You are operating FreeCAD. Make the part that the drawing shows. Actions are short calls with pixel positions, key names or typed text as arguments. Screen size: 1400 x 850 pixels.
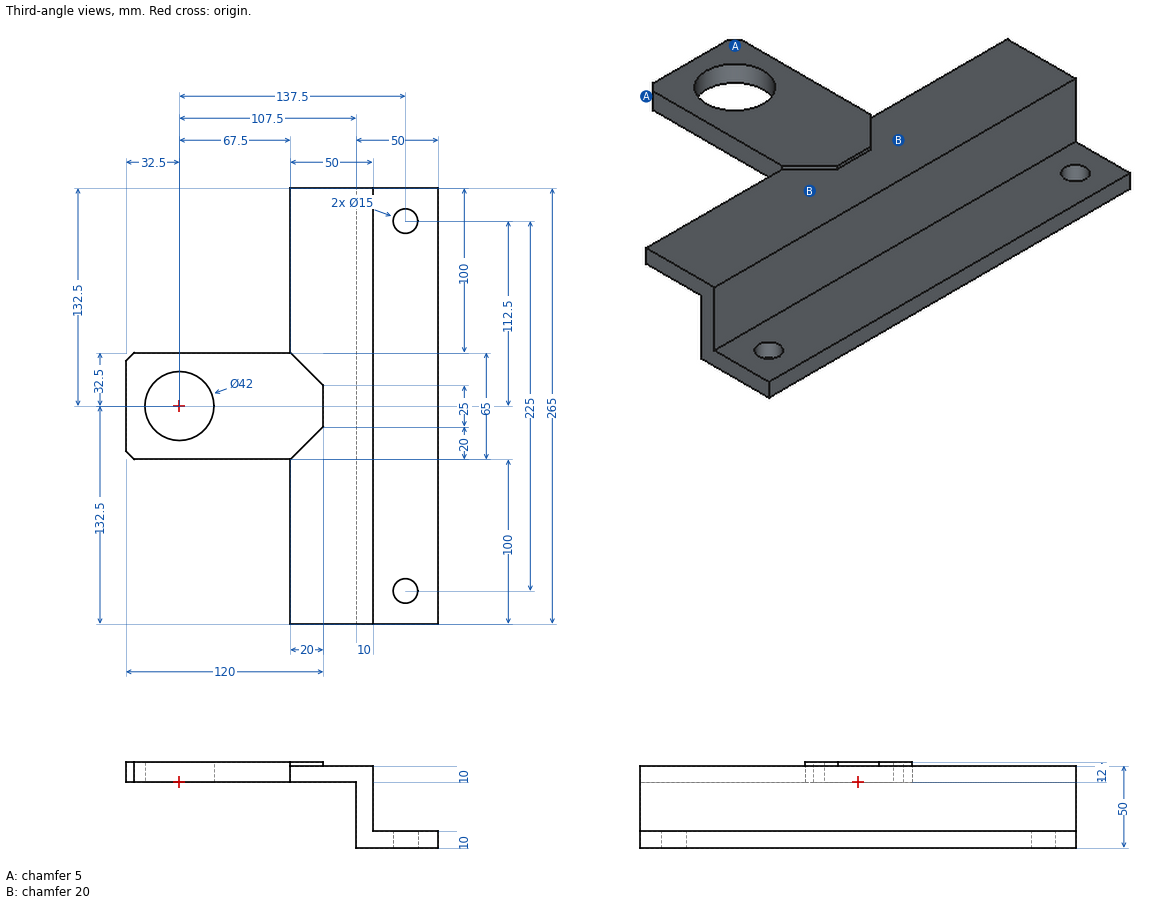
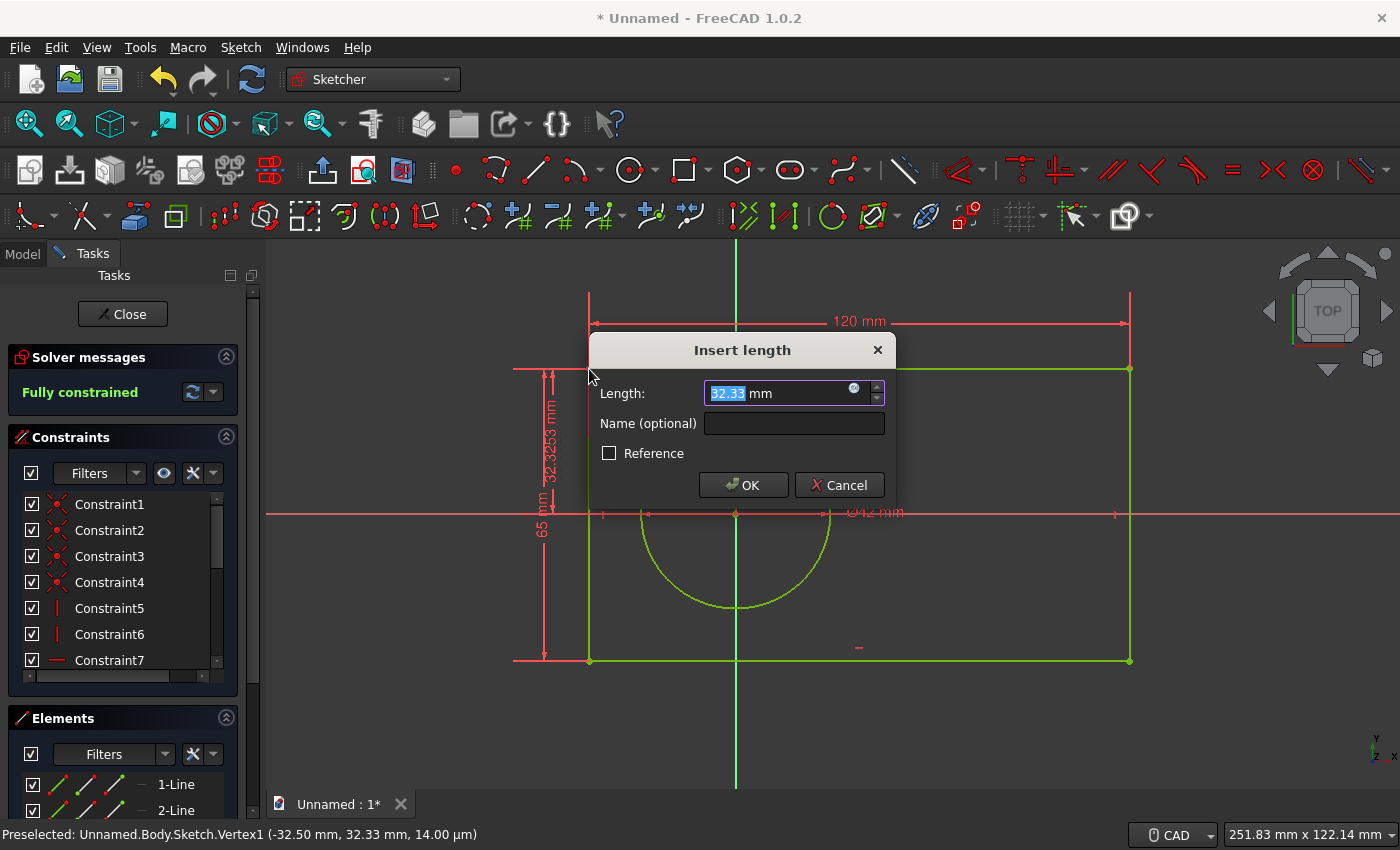
text(32.5)
key(Return)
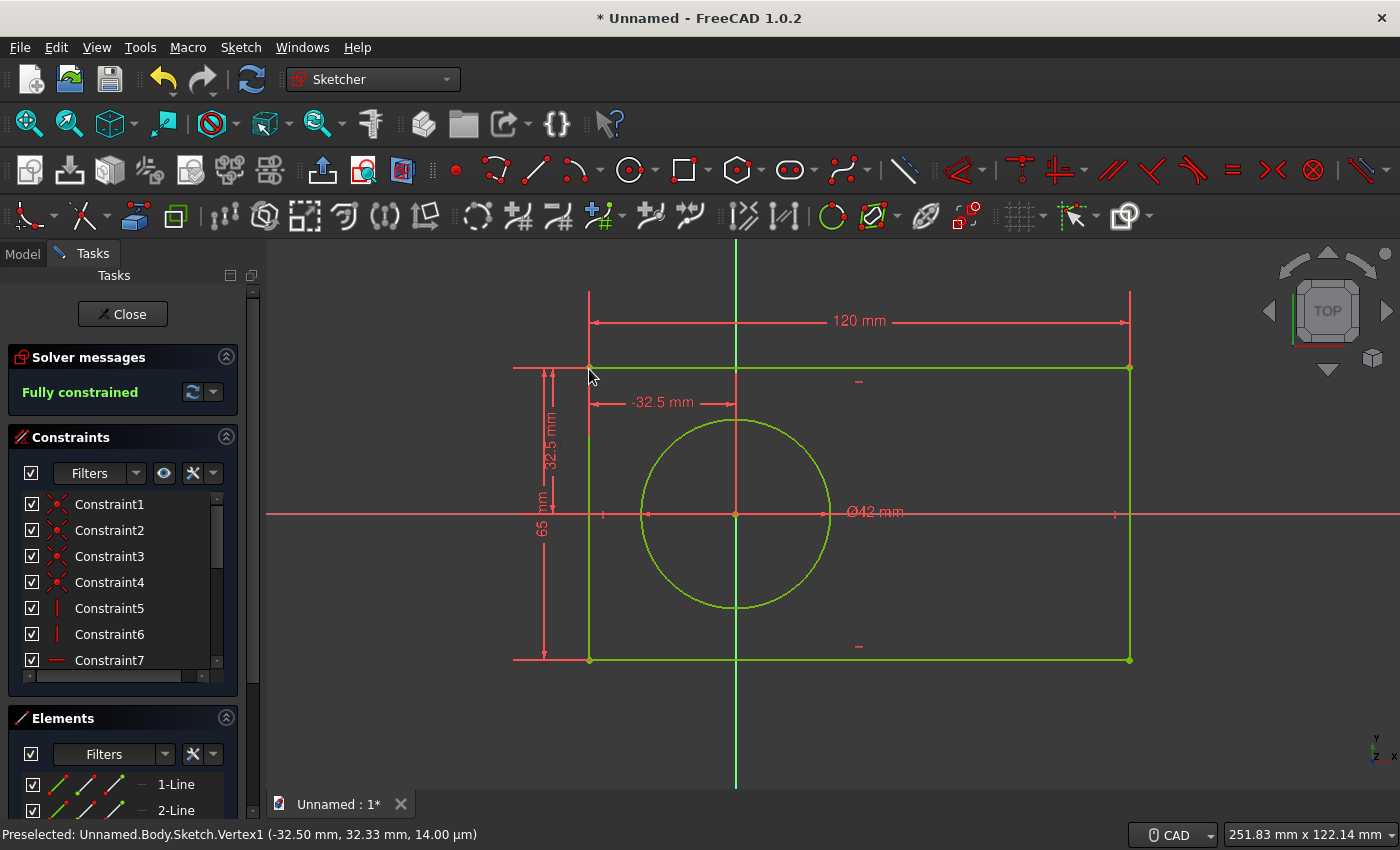
click(123, 314)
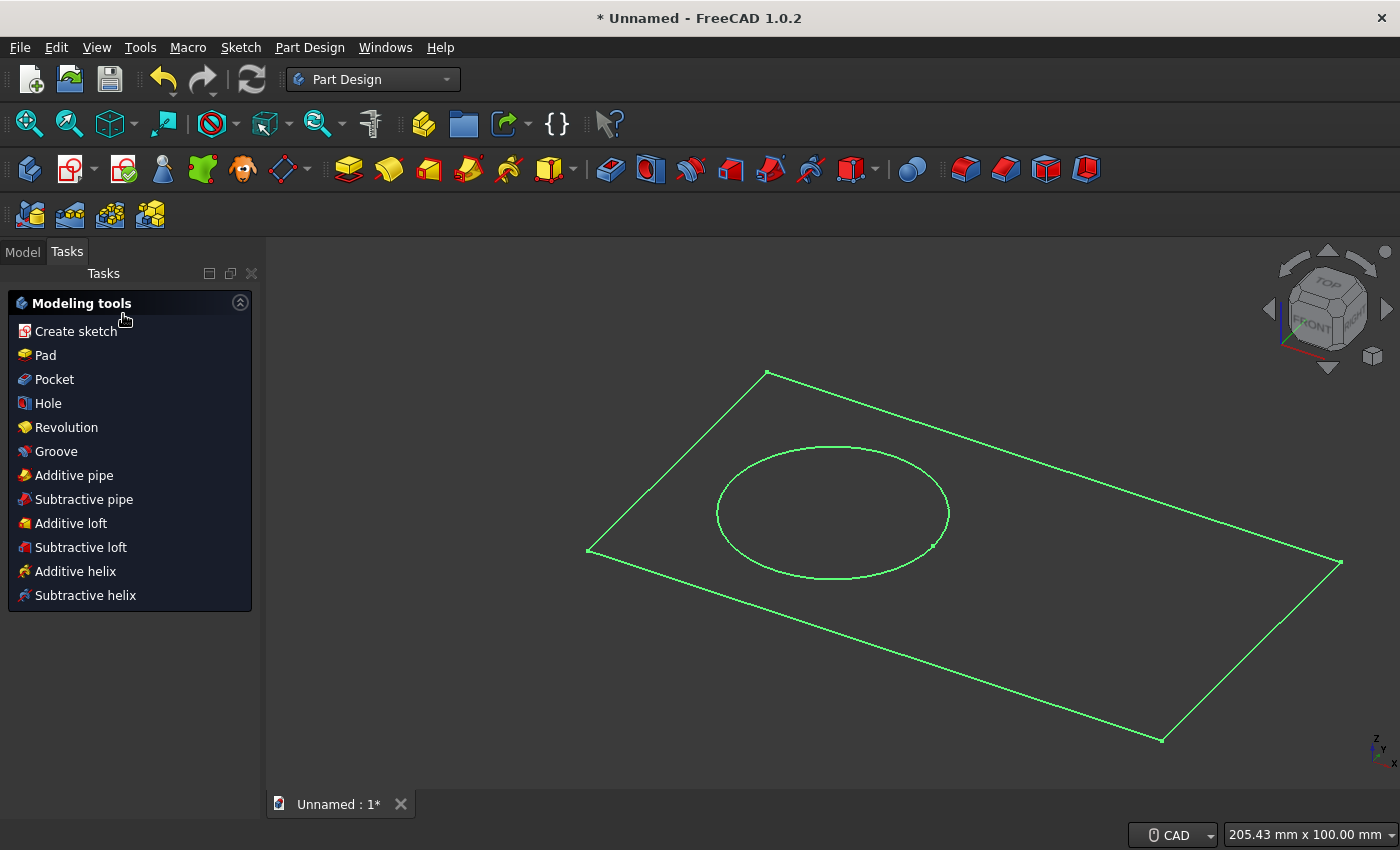
click(350, 170)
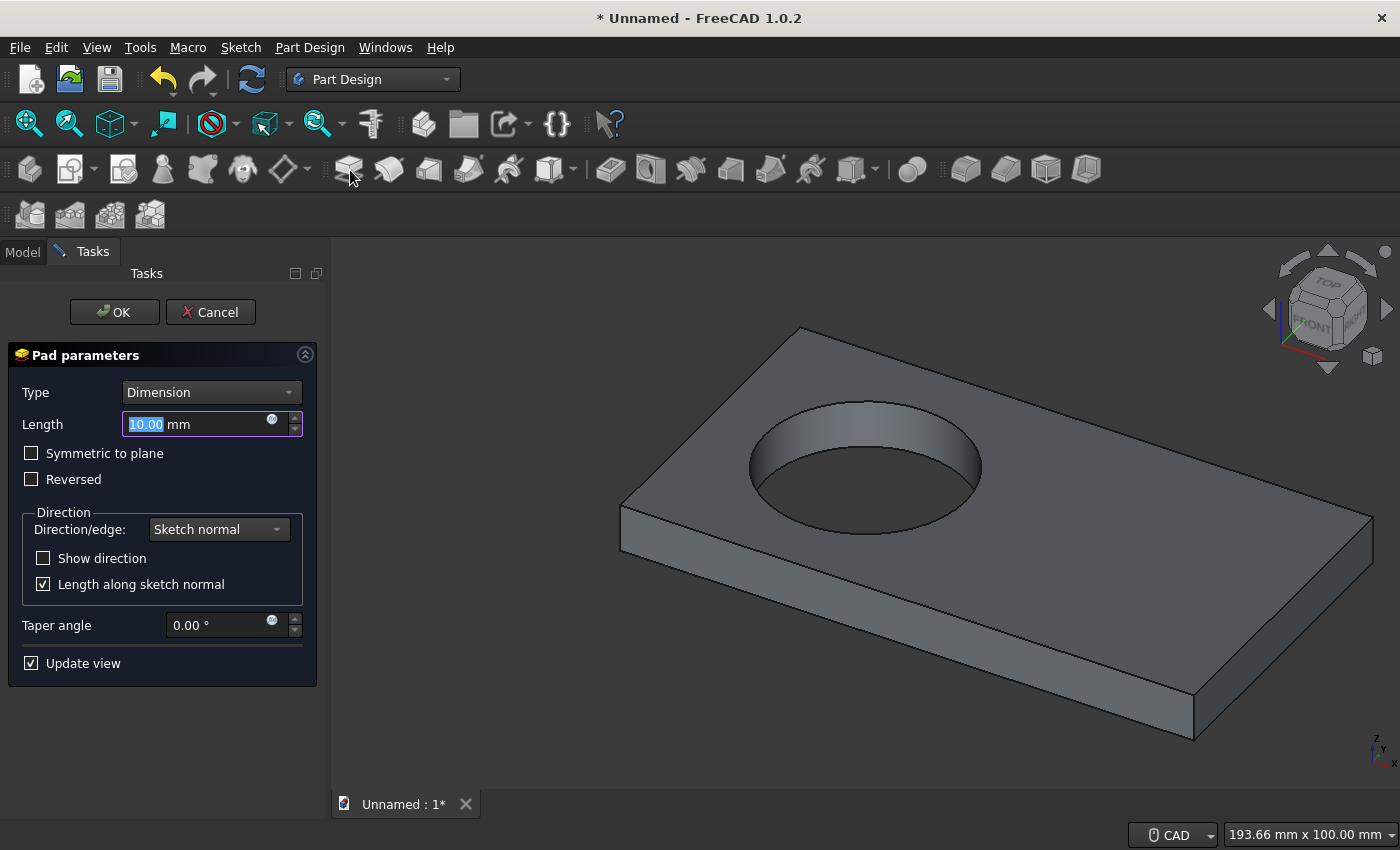
text(12)
key(Tab)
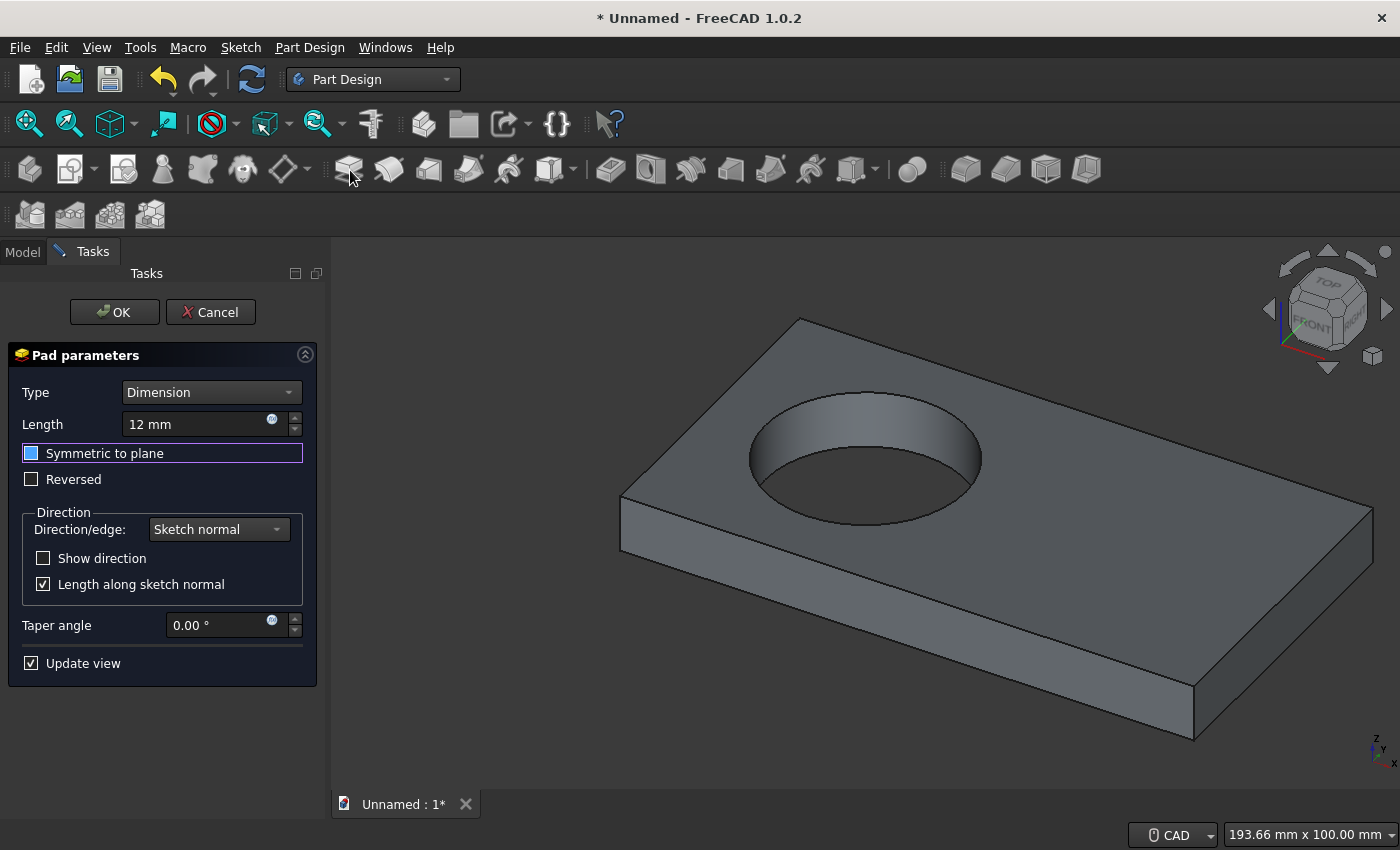
click(115, 312)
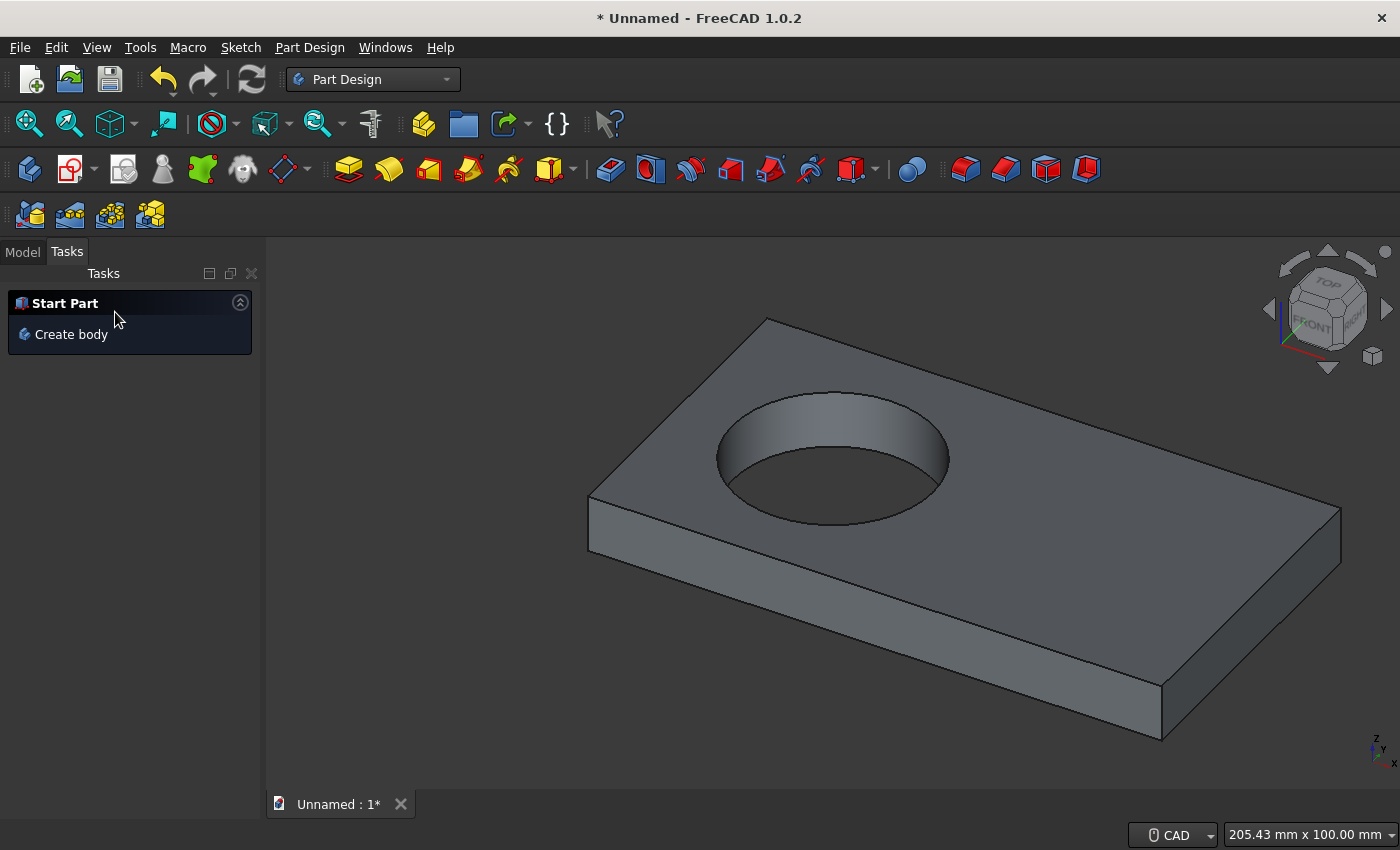
key(0)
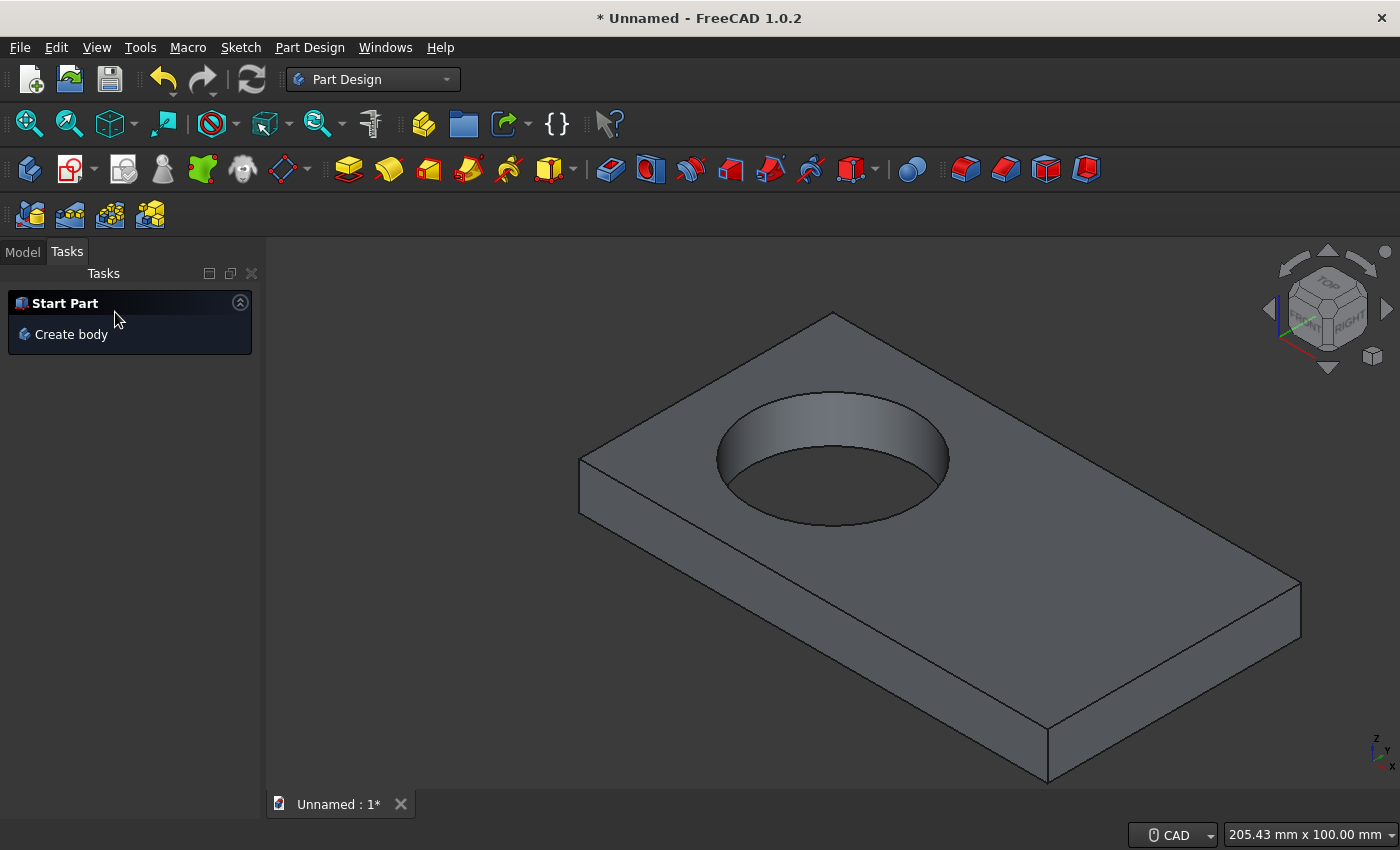
key(2)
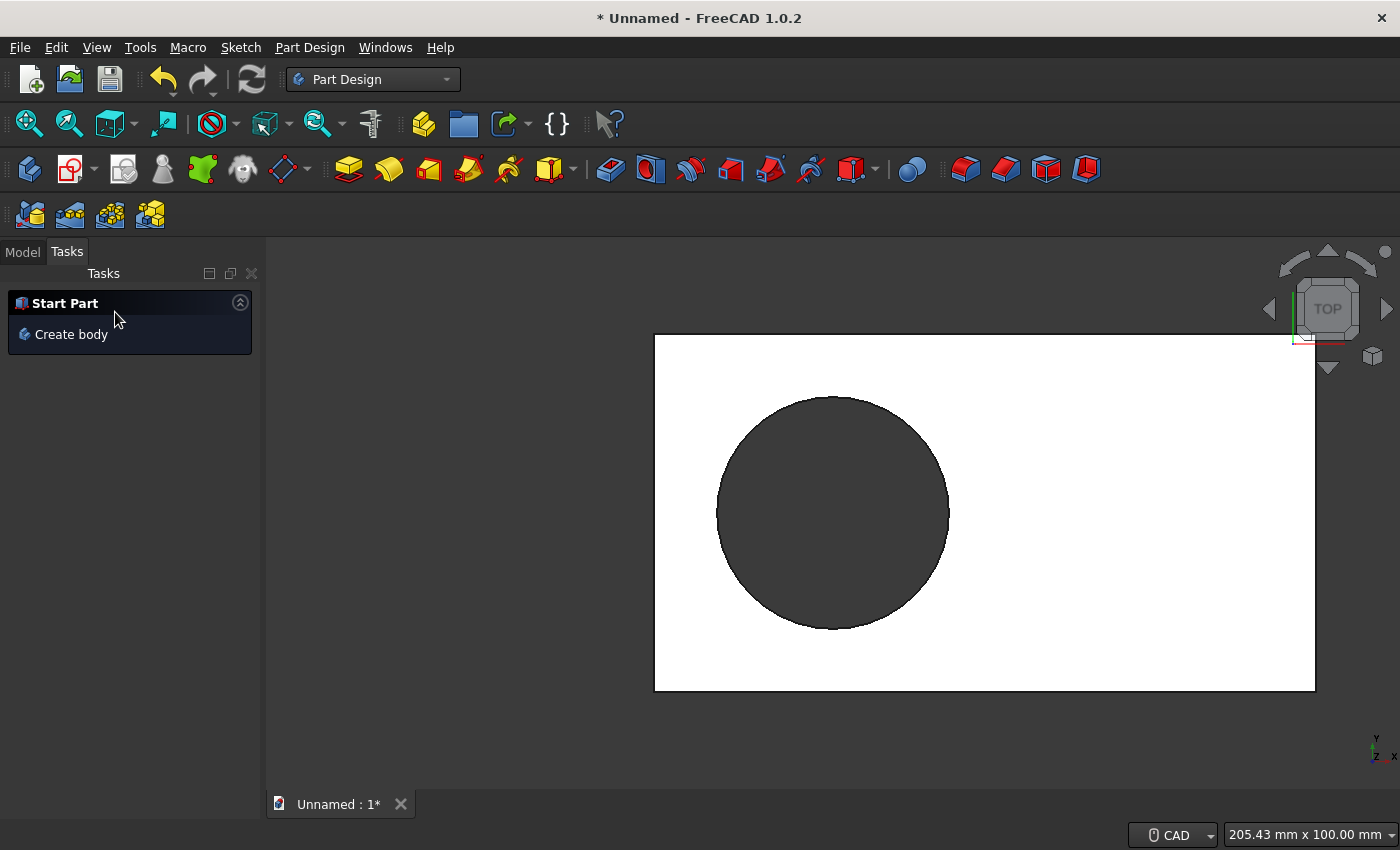
key(1)